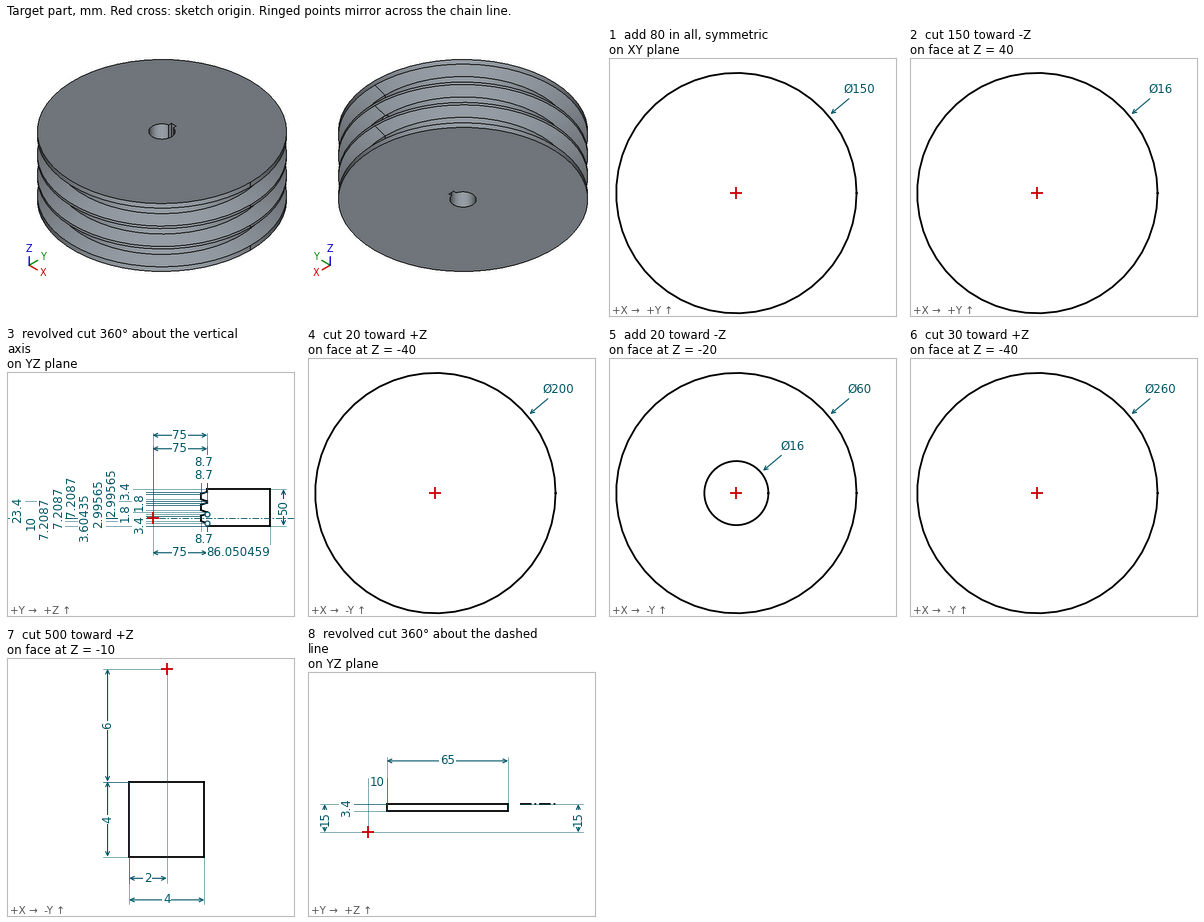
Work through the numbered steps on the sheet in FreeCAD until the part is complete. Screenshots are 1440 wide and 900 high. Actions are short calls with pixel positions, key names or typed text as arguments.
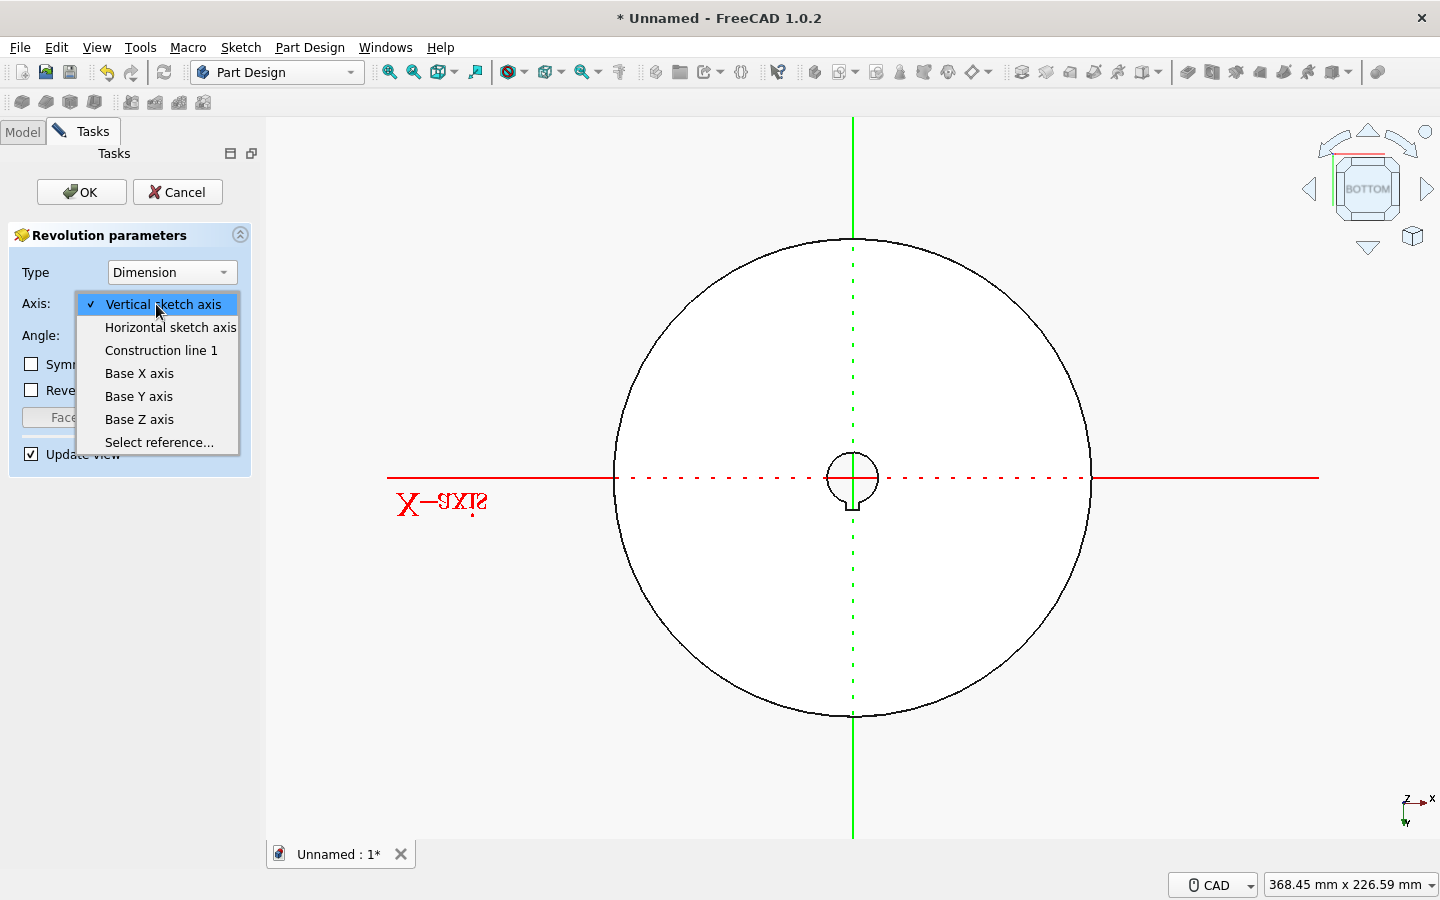
click(156, 350)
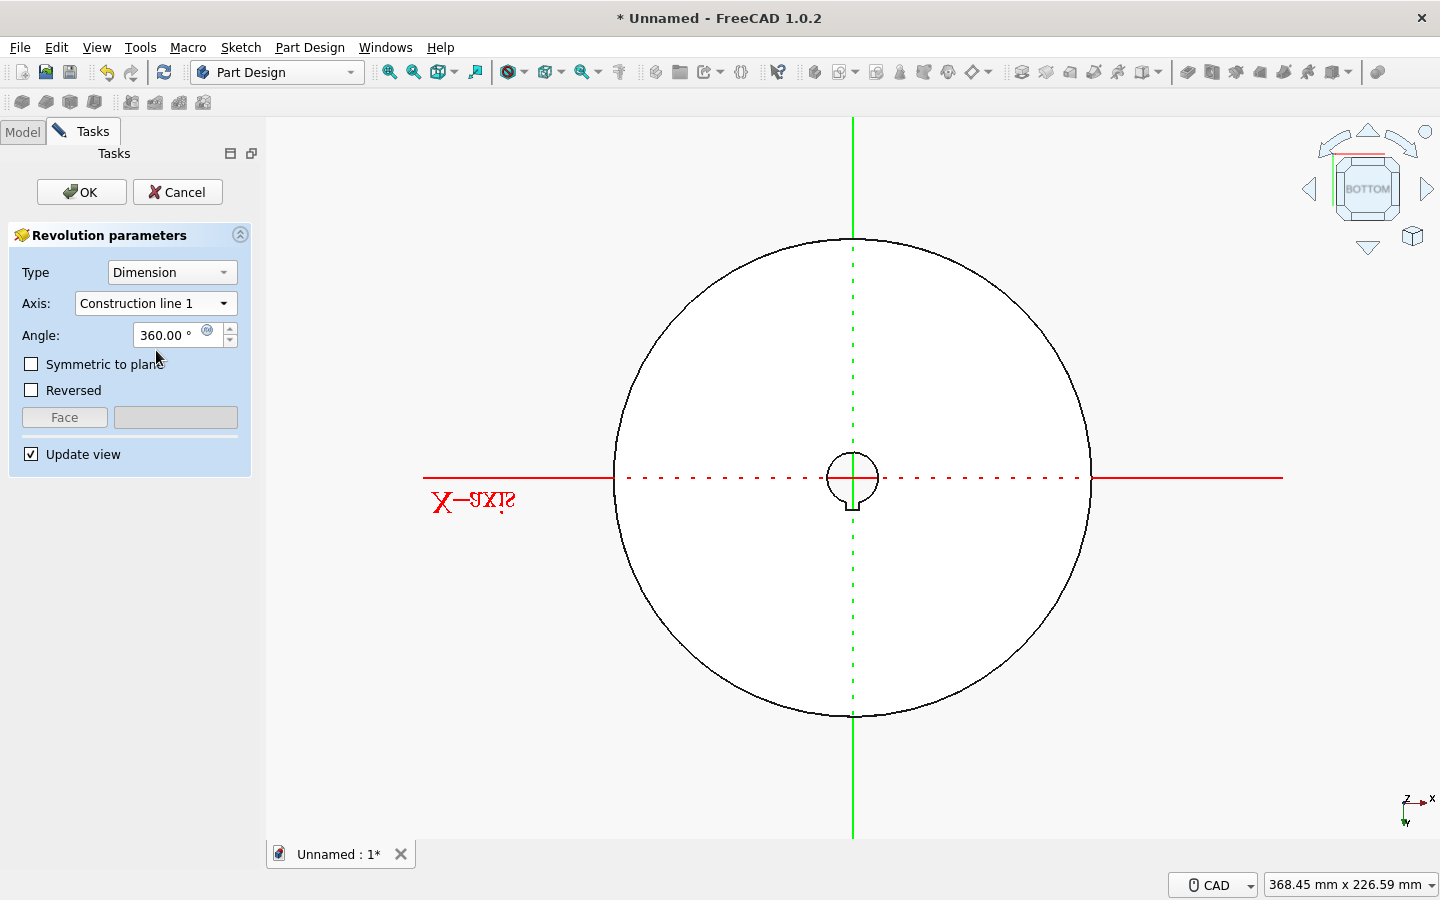
click(82, 192)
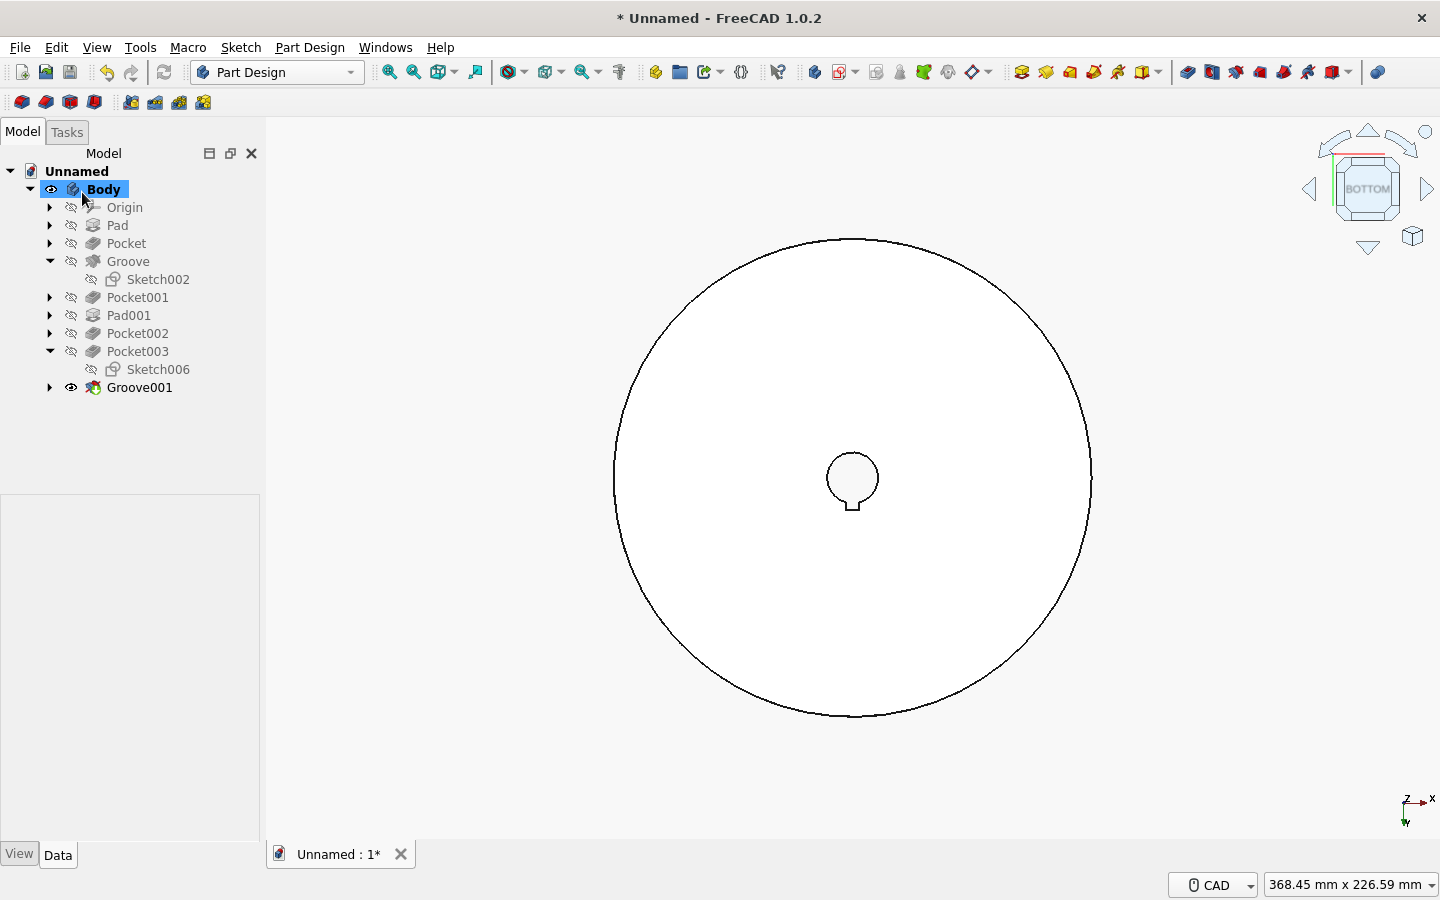
key(0)